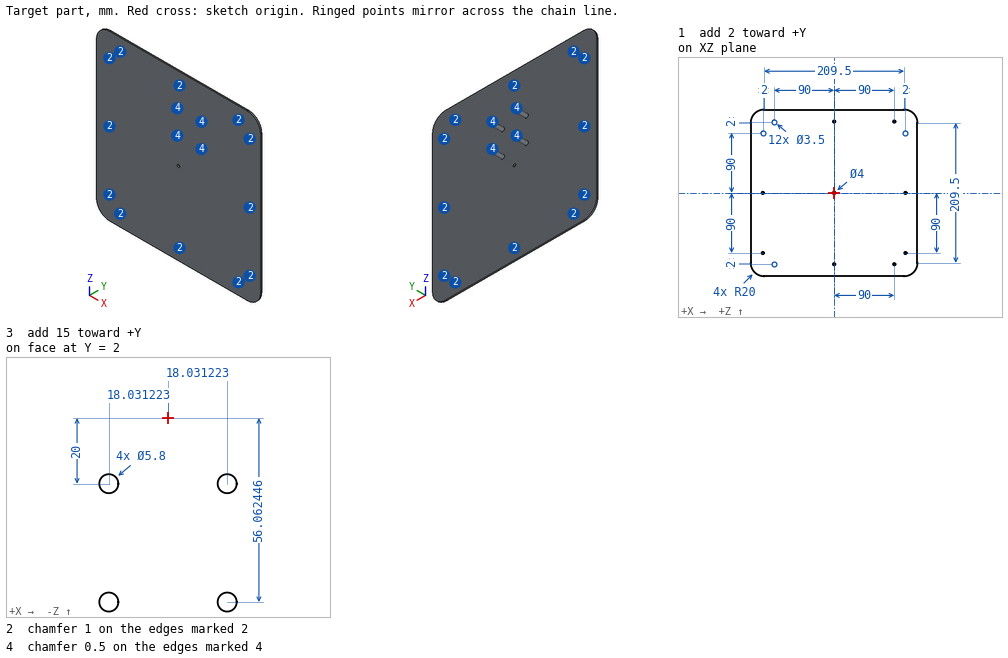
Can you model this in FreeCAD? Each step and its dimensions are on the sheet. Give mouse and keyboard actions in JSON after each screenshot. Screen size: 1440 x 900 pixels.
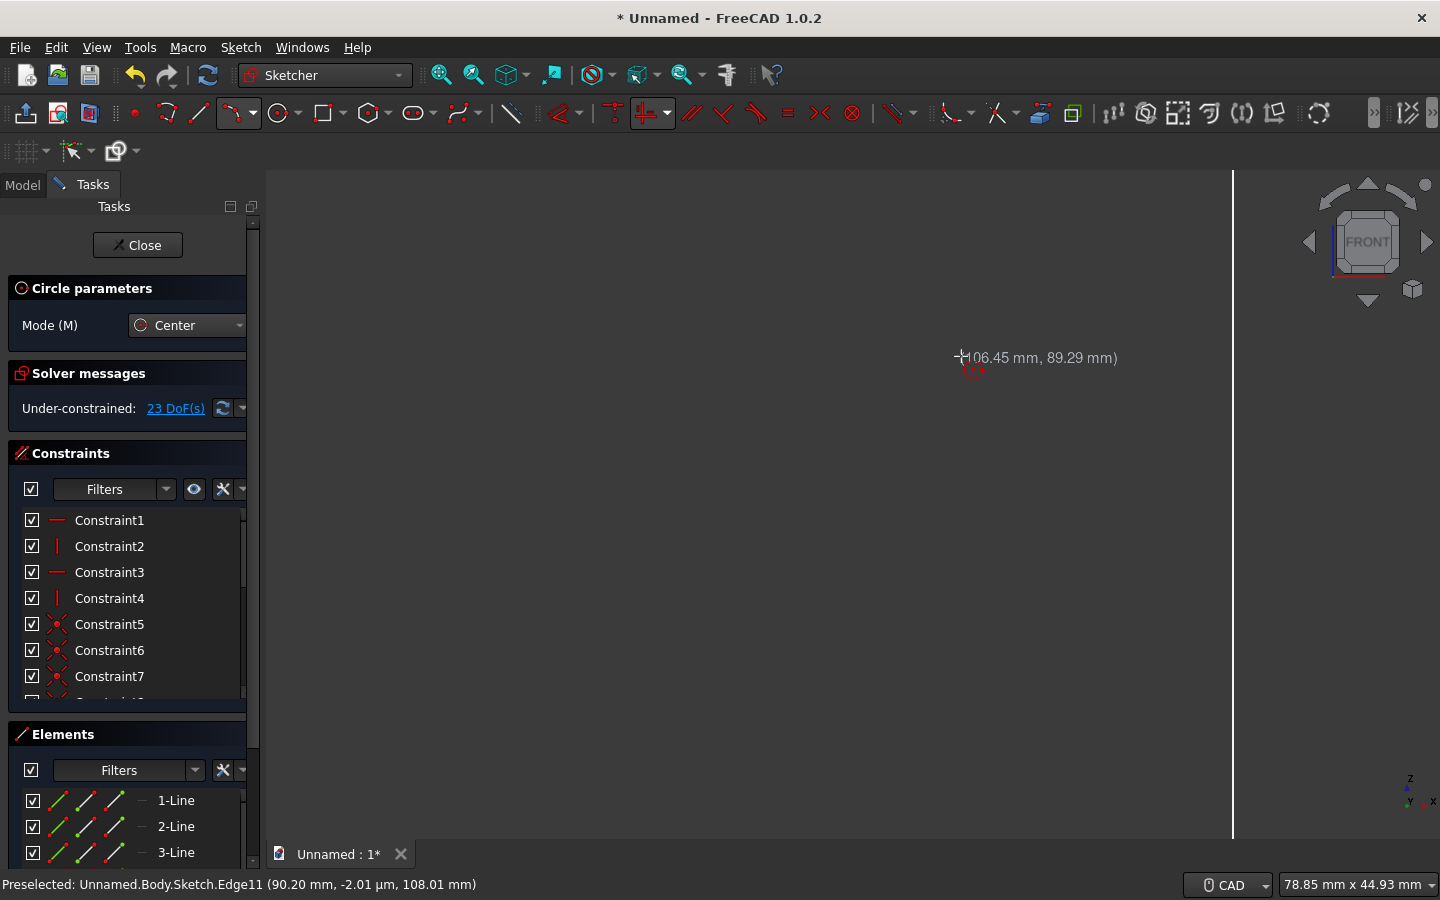
{"action": "scroll", "coordinate": [961, 357], "scroll_direction": "down", "scroll_amount": 11}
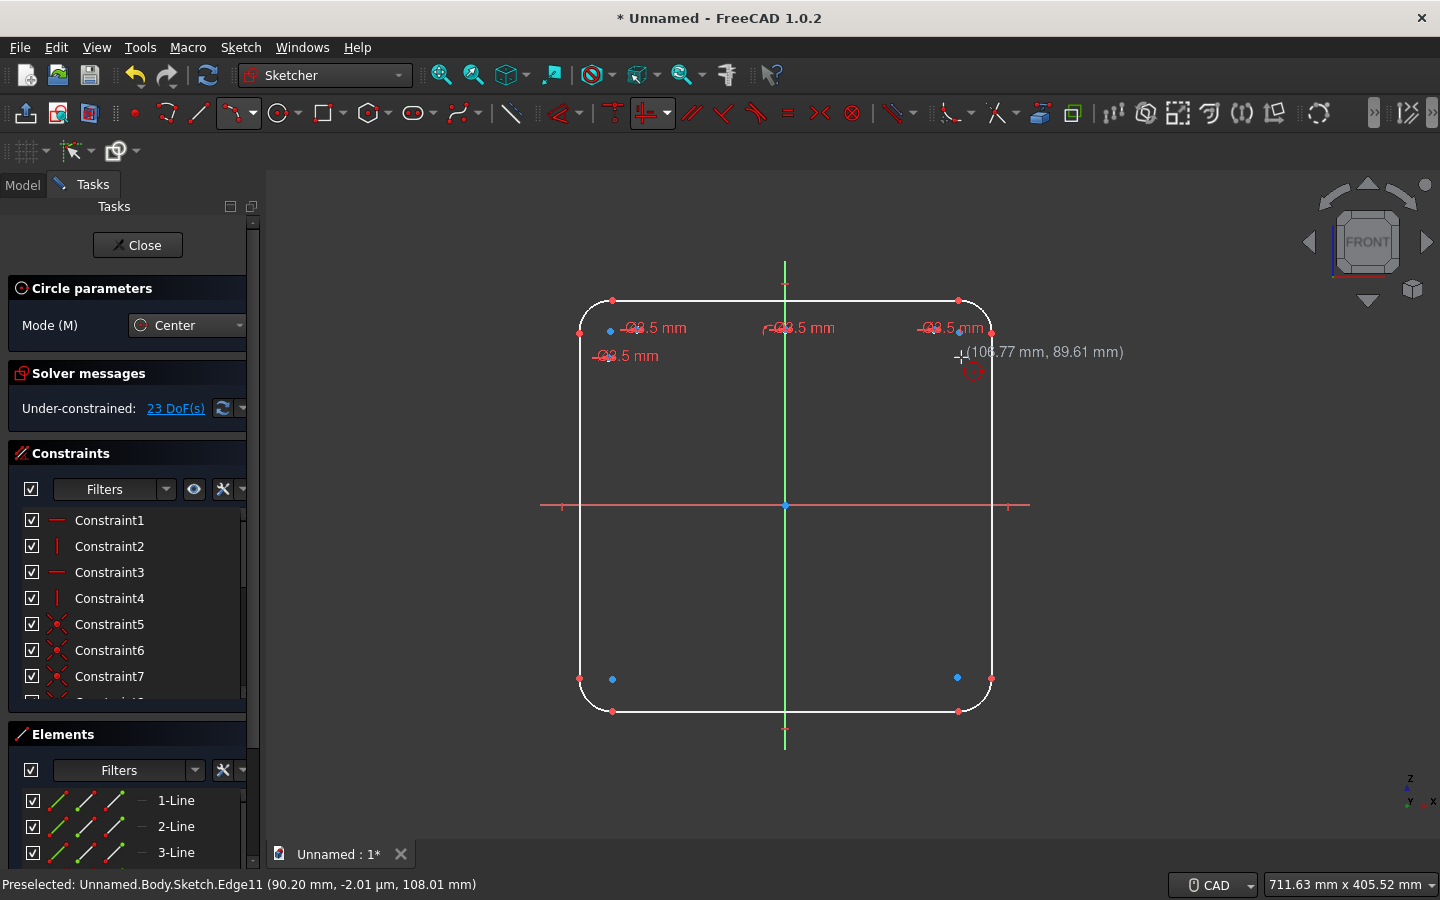
{"action": "left_click", "coordinate": [961, 357]}
{"action": "mouse_move", "coordinate": [964, 355]}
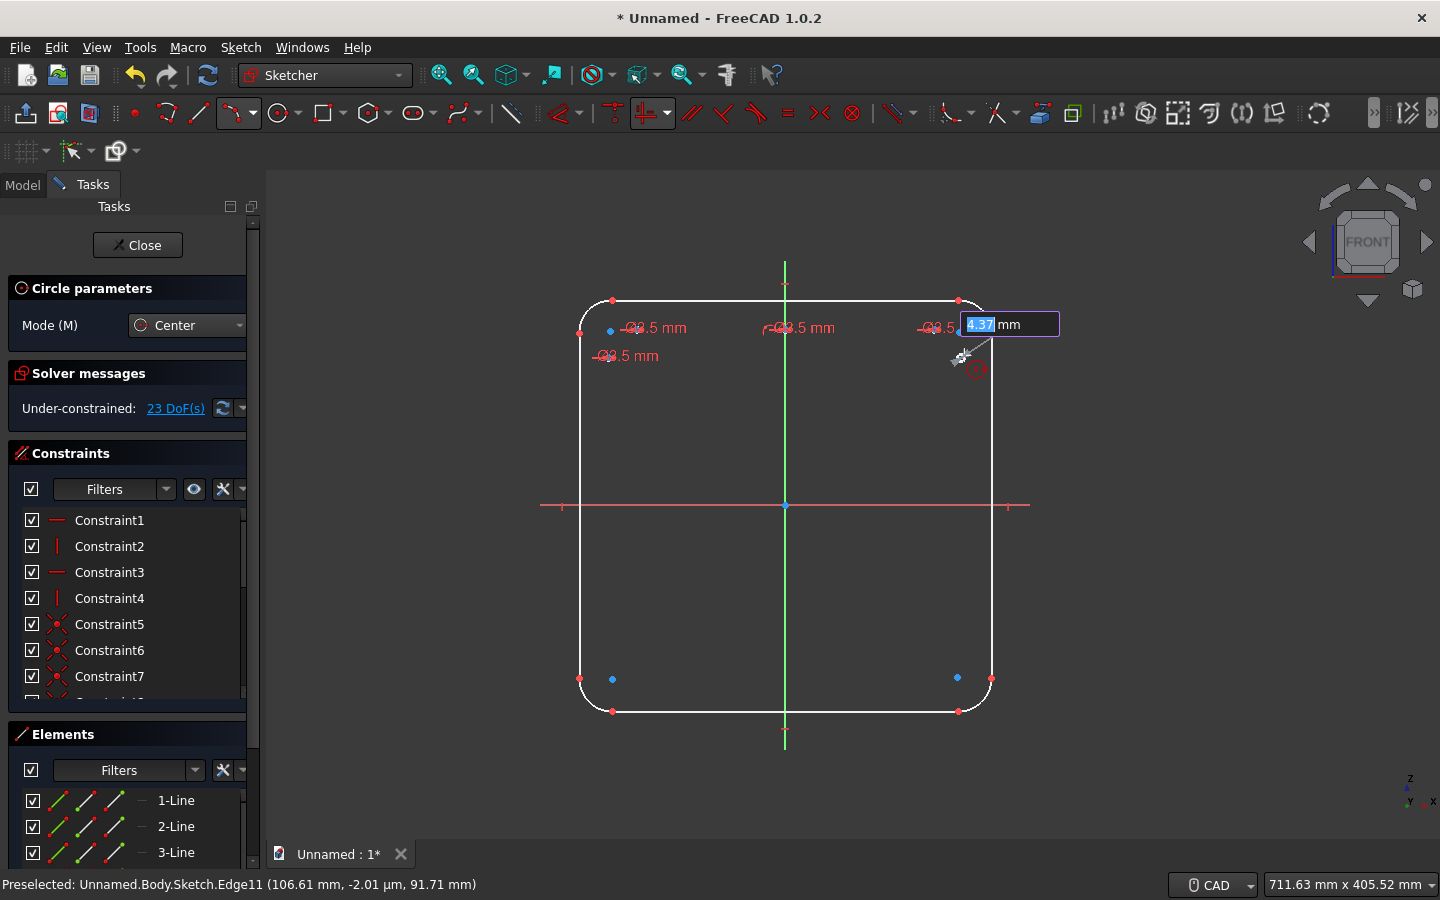
{"action": "type", "text": "3.5"}
{"action": "key", "text": "Return"}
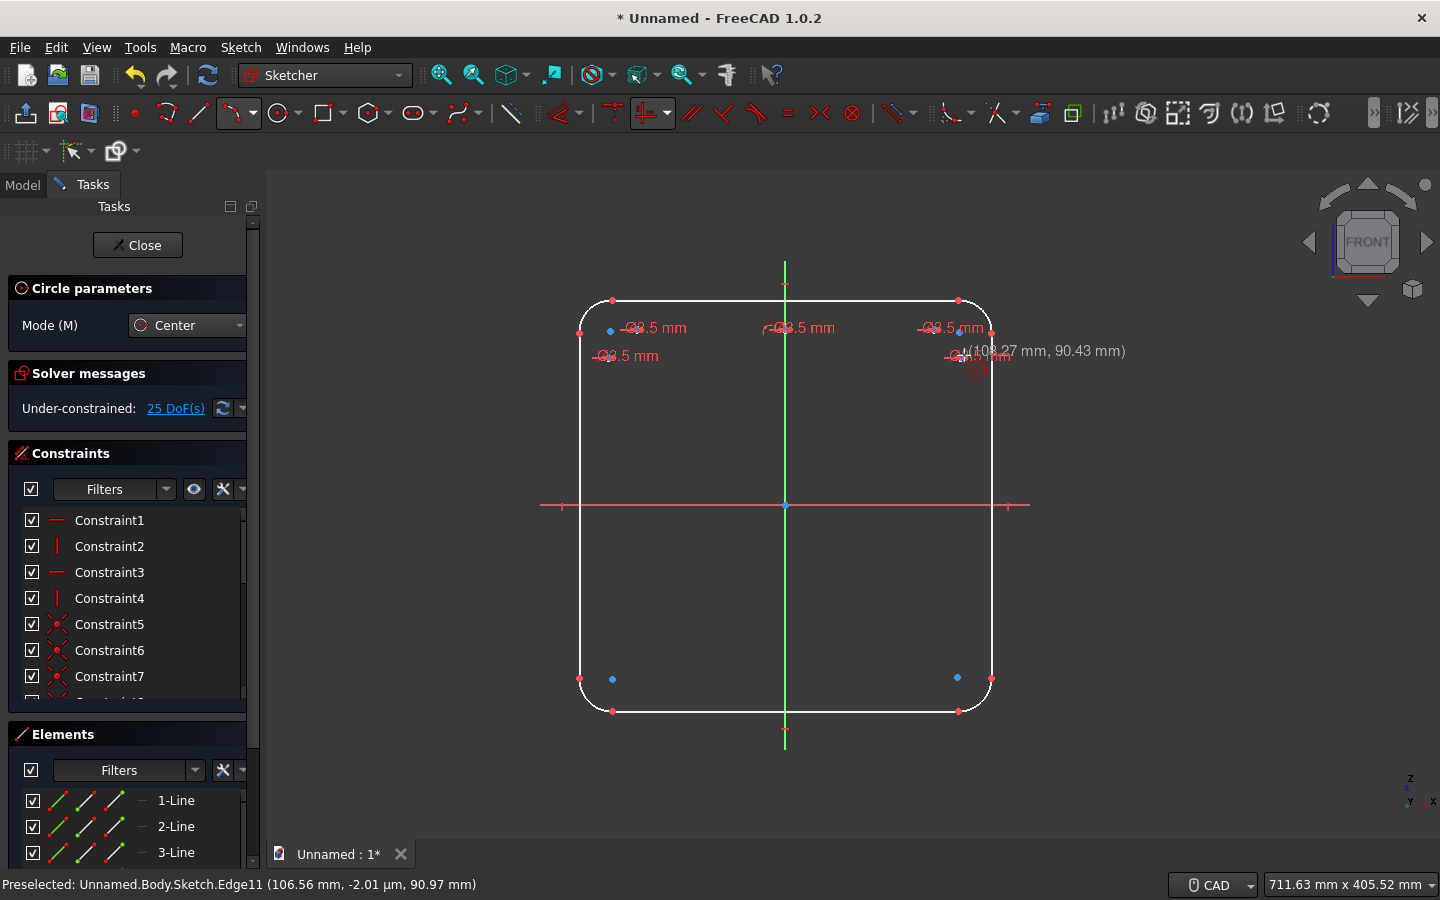
{"action": "scroll", "coordinate": [609, 505], "scroll_direction": "up", "scroll_amount": 11}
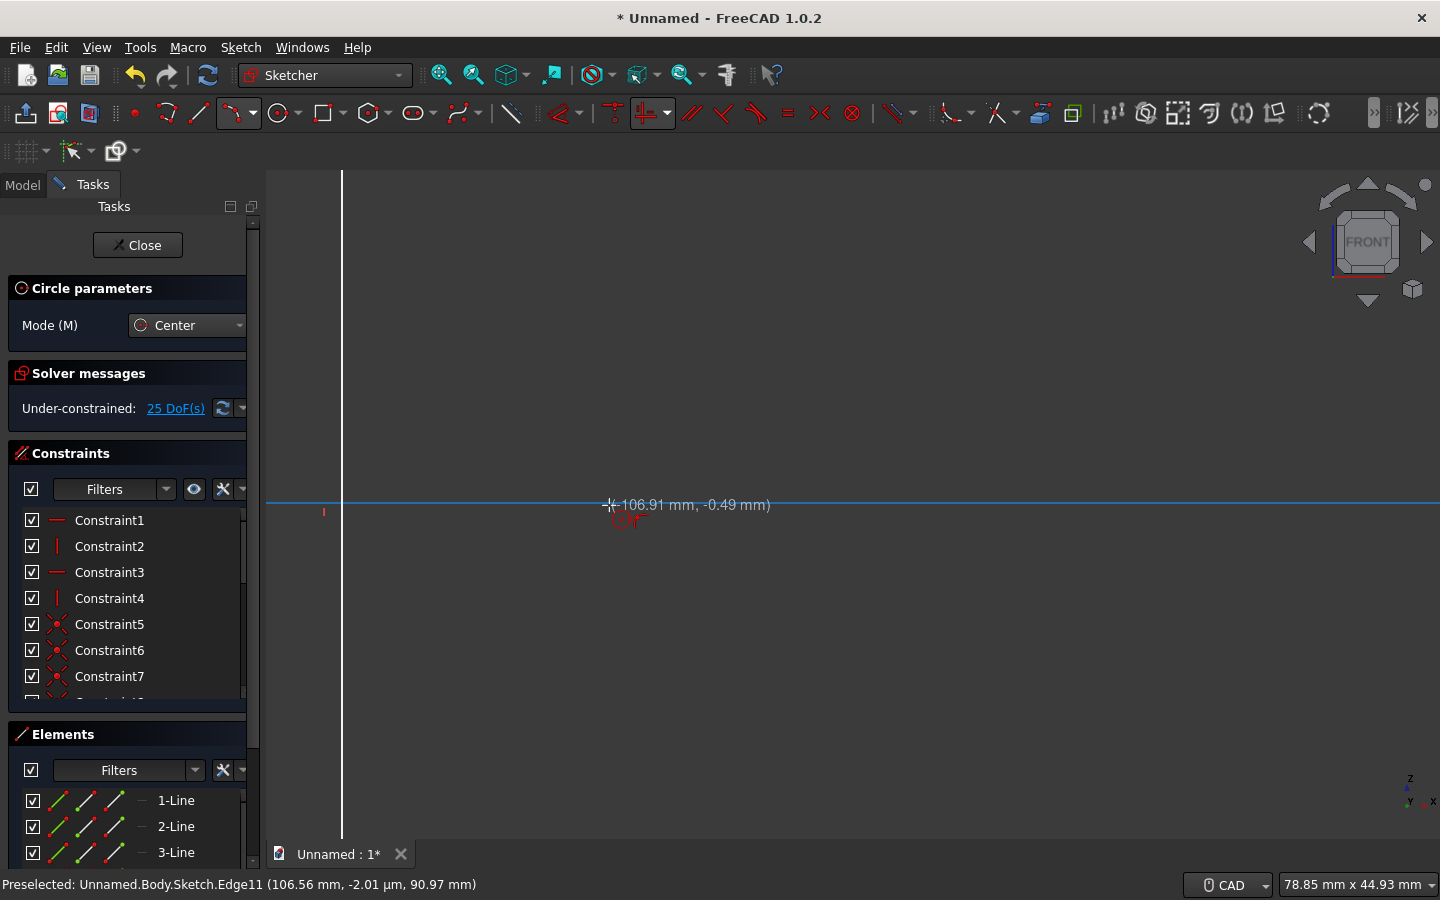
{"action": "scroll", "coordinate": [608, 505], "scroll_direction": "down", "scroll_amount": 11}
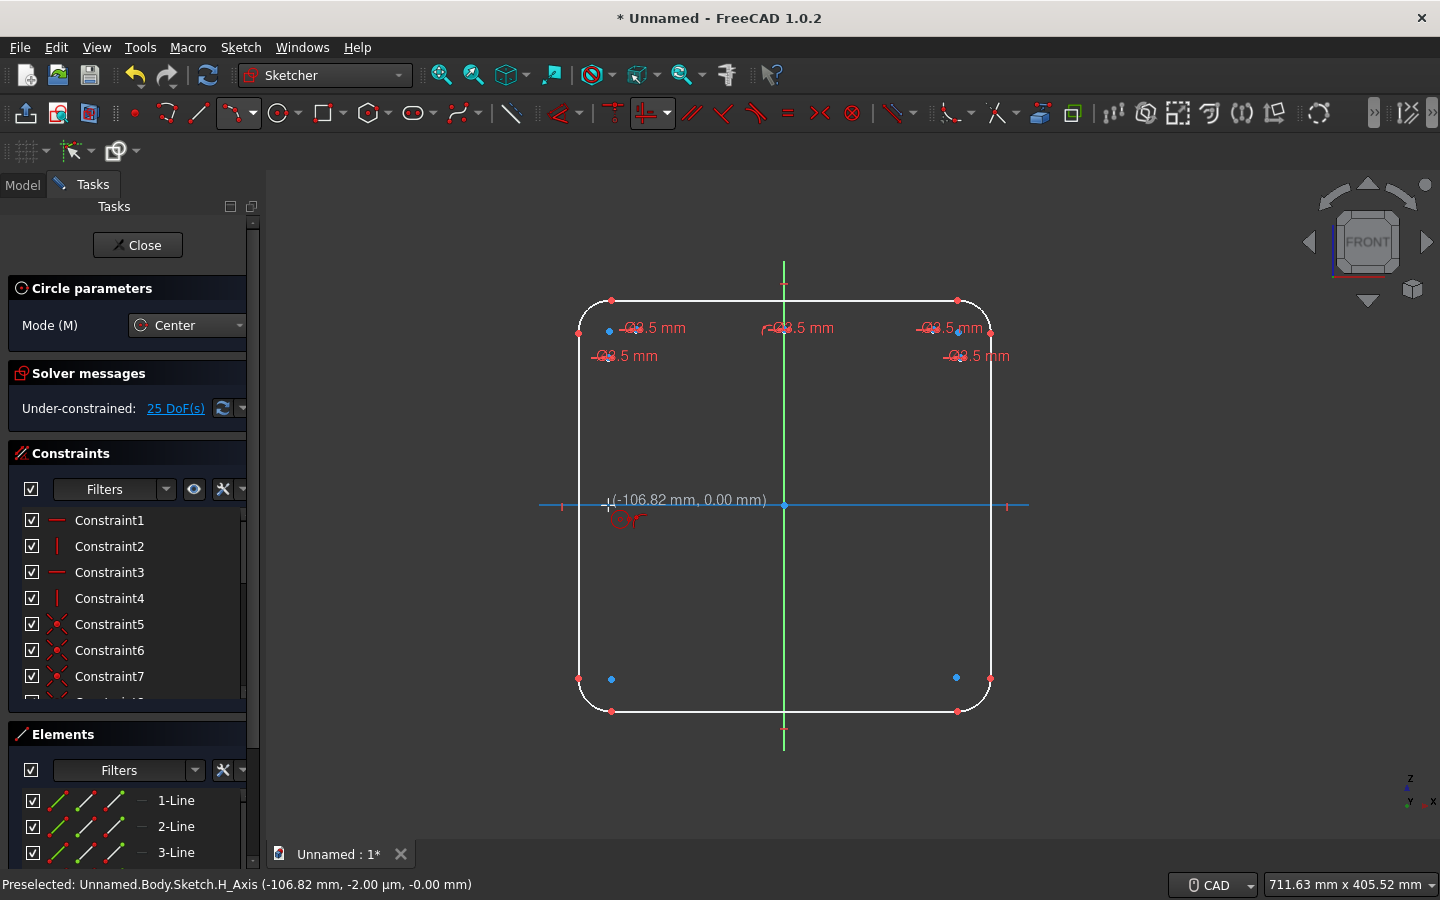
{"action": "left_click", "coordinate": [608, 505]}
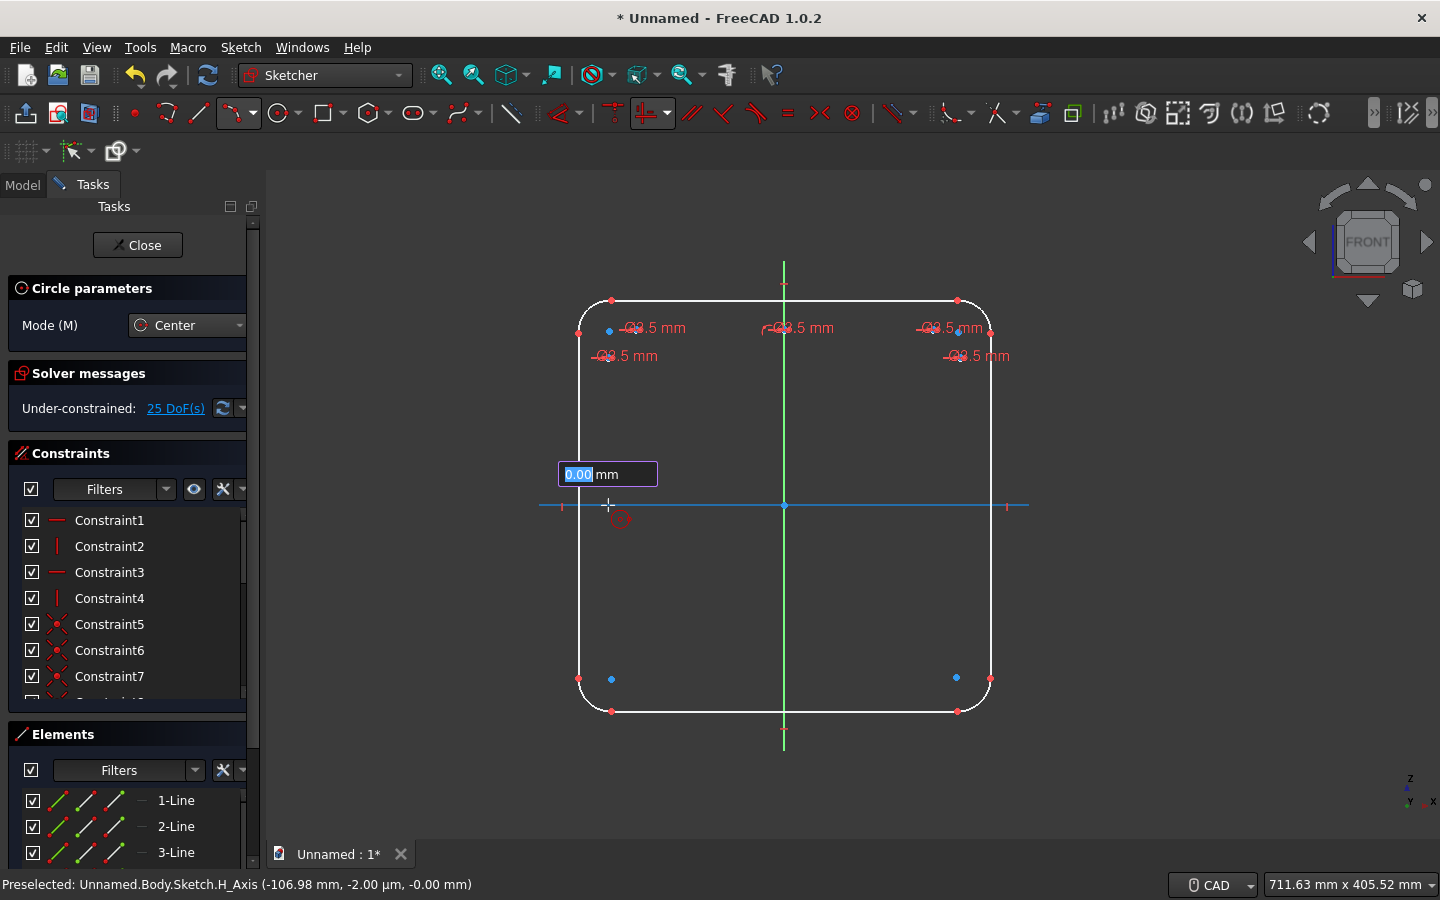
{"action": "scroll", "coordinate": [609, 502], "scroll_direction": "up", "scroll_amount": 9}
{"action": "mouse_move", "coordinate": [610, 502]}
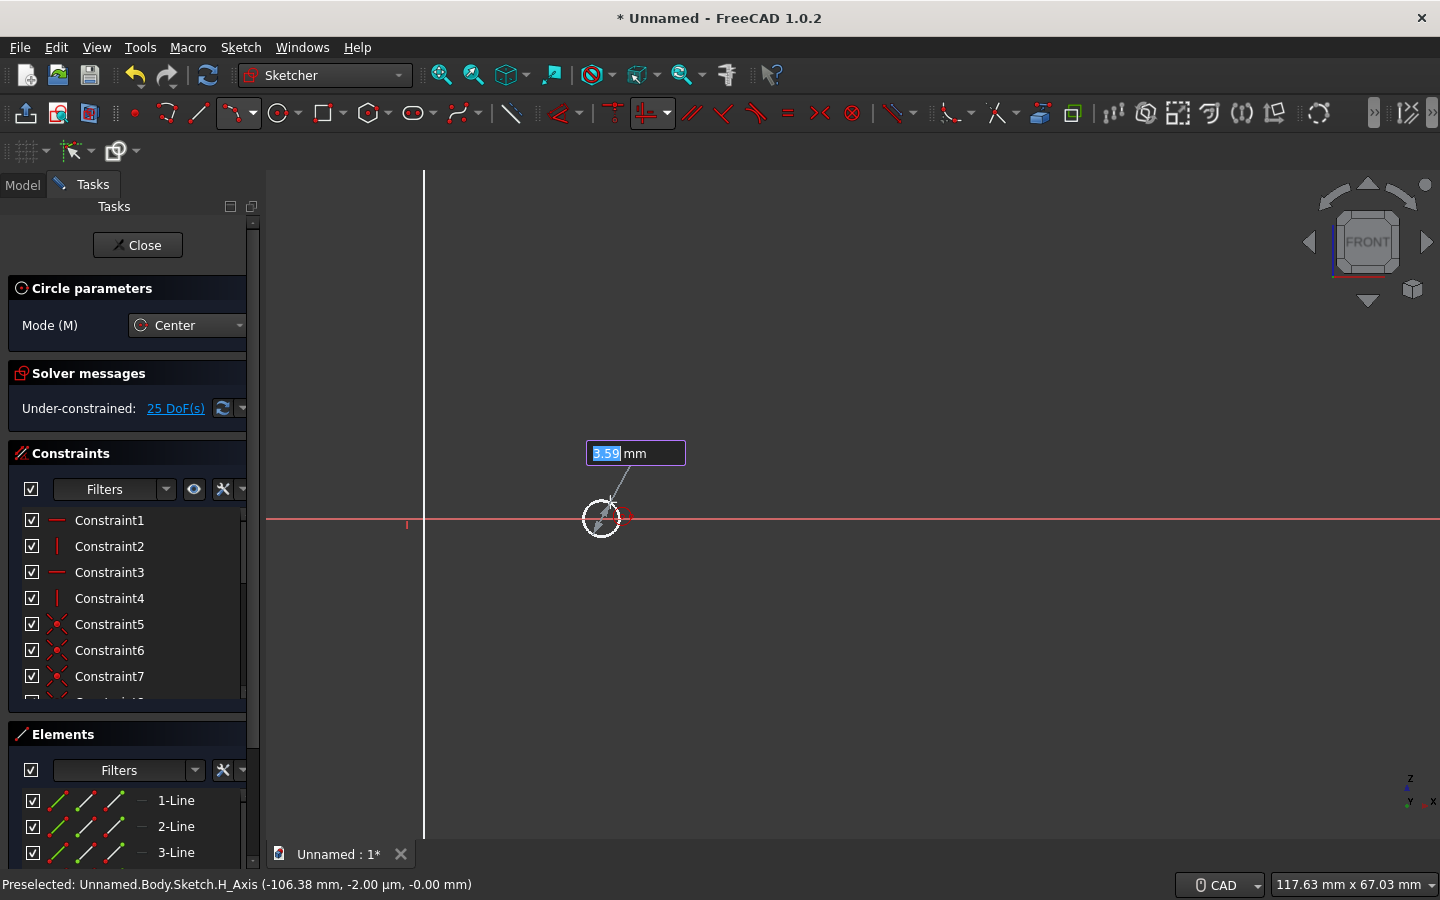
{"action": "type", "text": "3.5"}
{"action": "key", "text": "Return"}